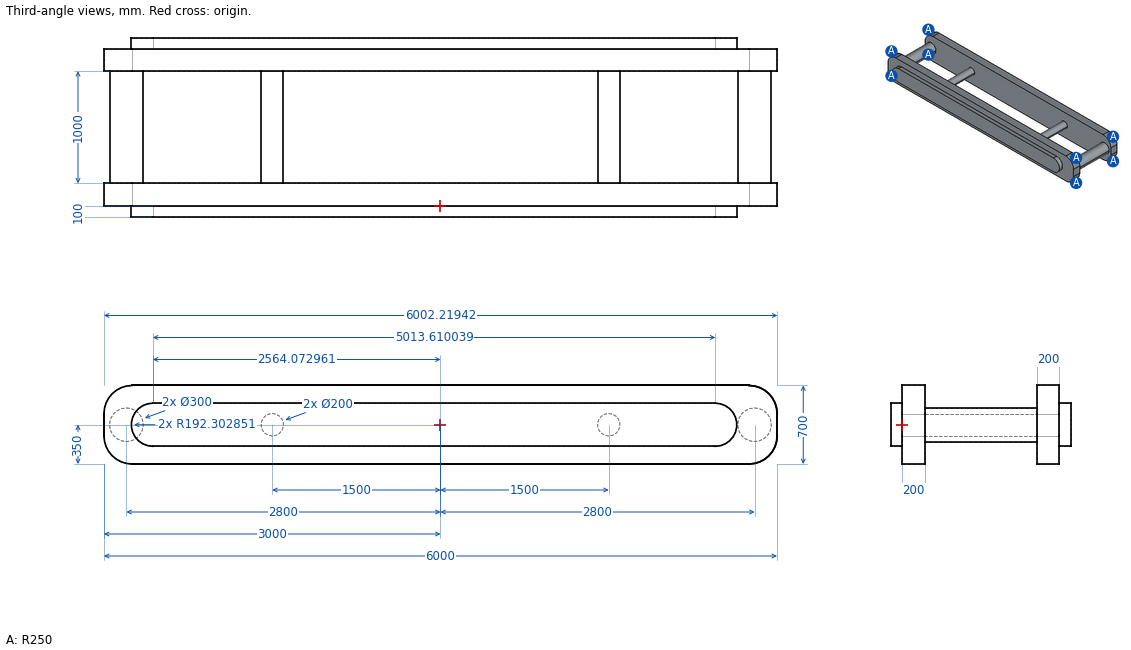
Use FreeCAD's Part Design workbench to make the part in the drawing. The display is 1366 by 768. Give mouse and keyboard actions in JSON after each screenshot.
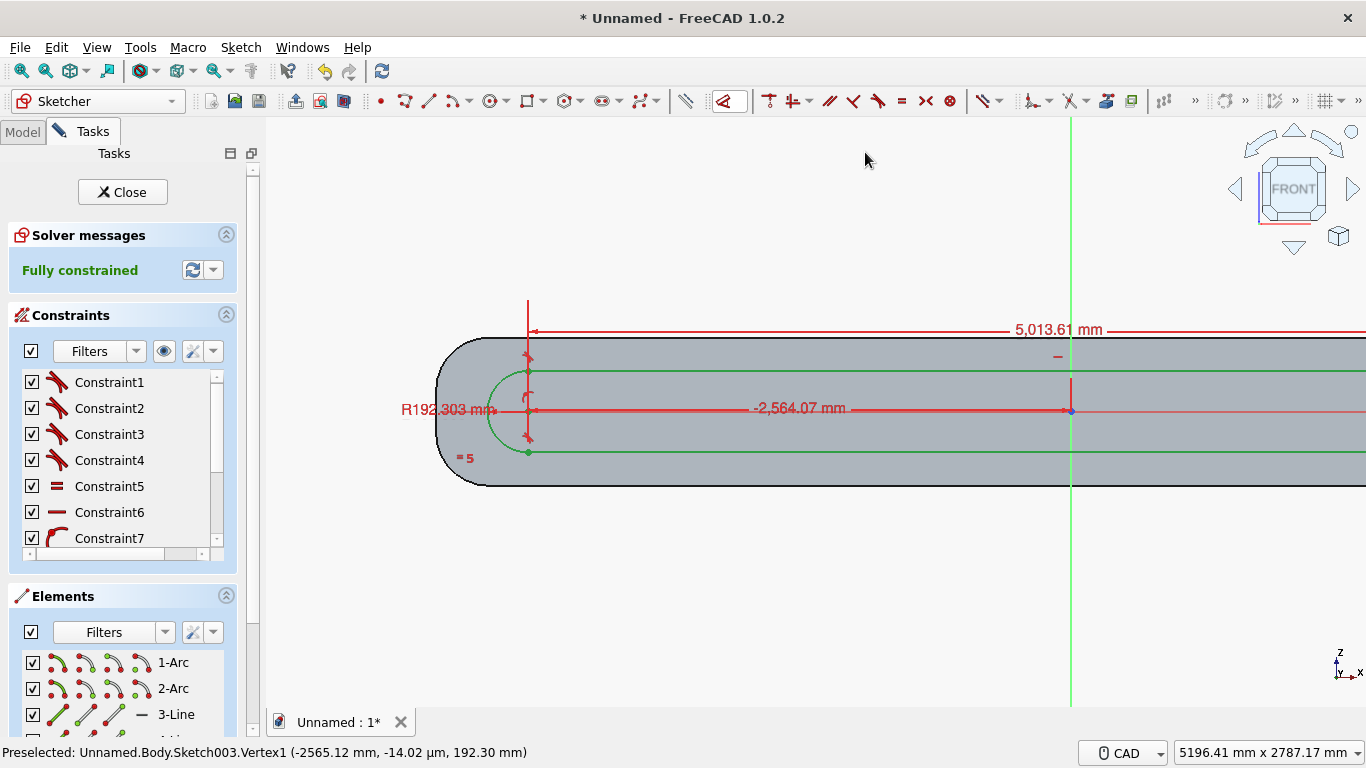
{"action": "left_click", "coordinate": [123, 192]}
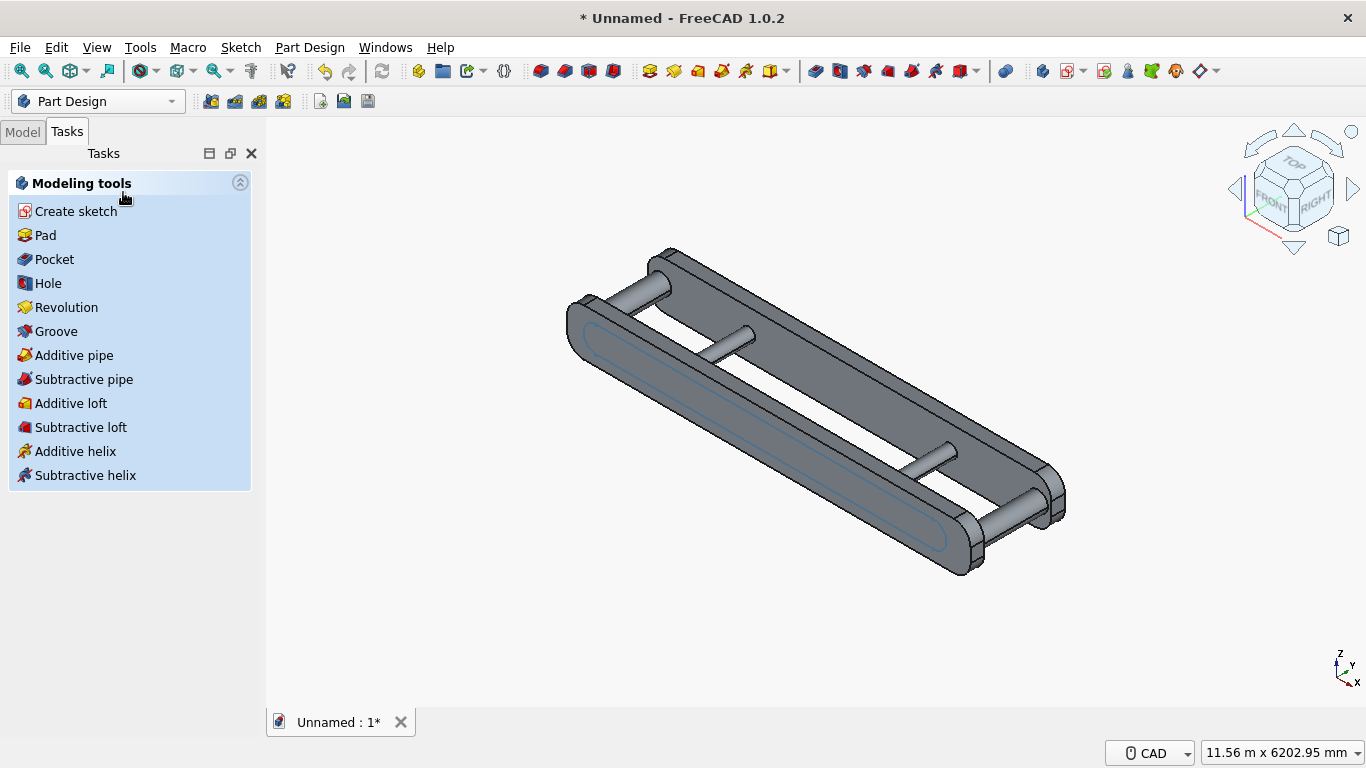
{"action": "left_click", "coordinate": [650, 72]}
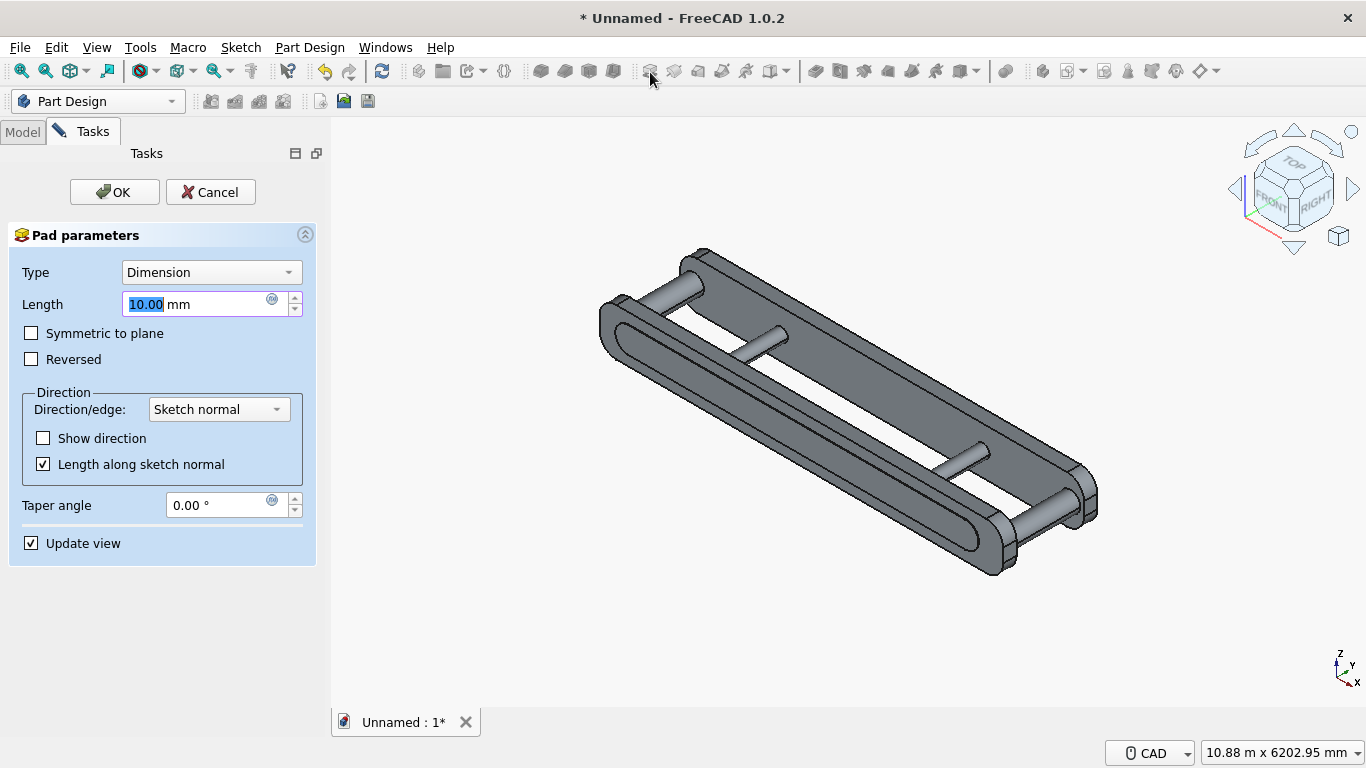
{"action": "type", "text": "100"}
{"action": "key", "text": "Tab"}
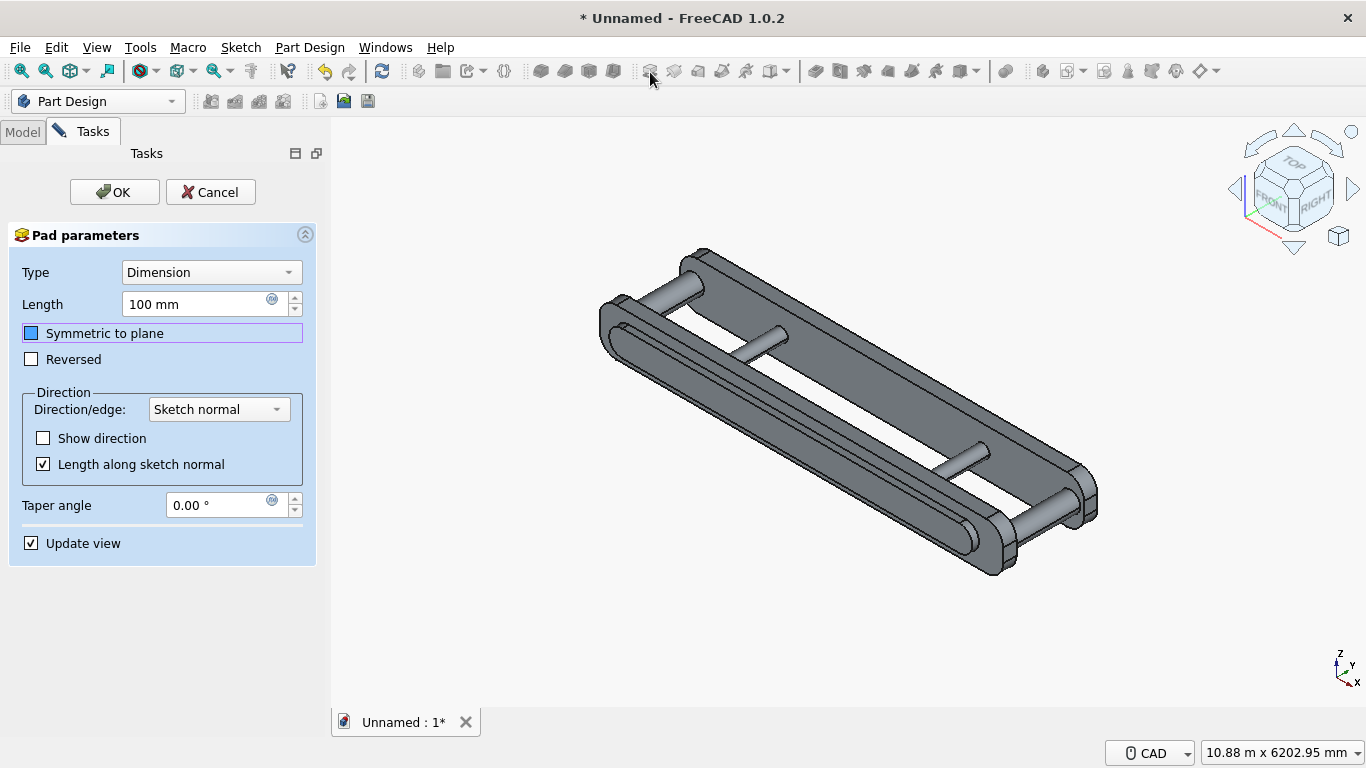
{"action": "left_click", "coordinate": [115, 192]}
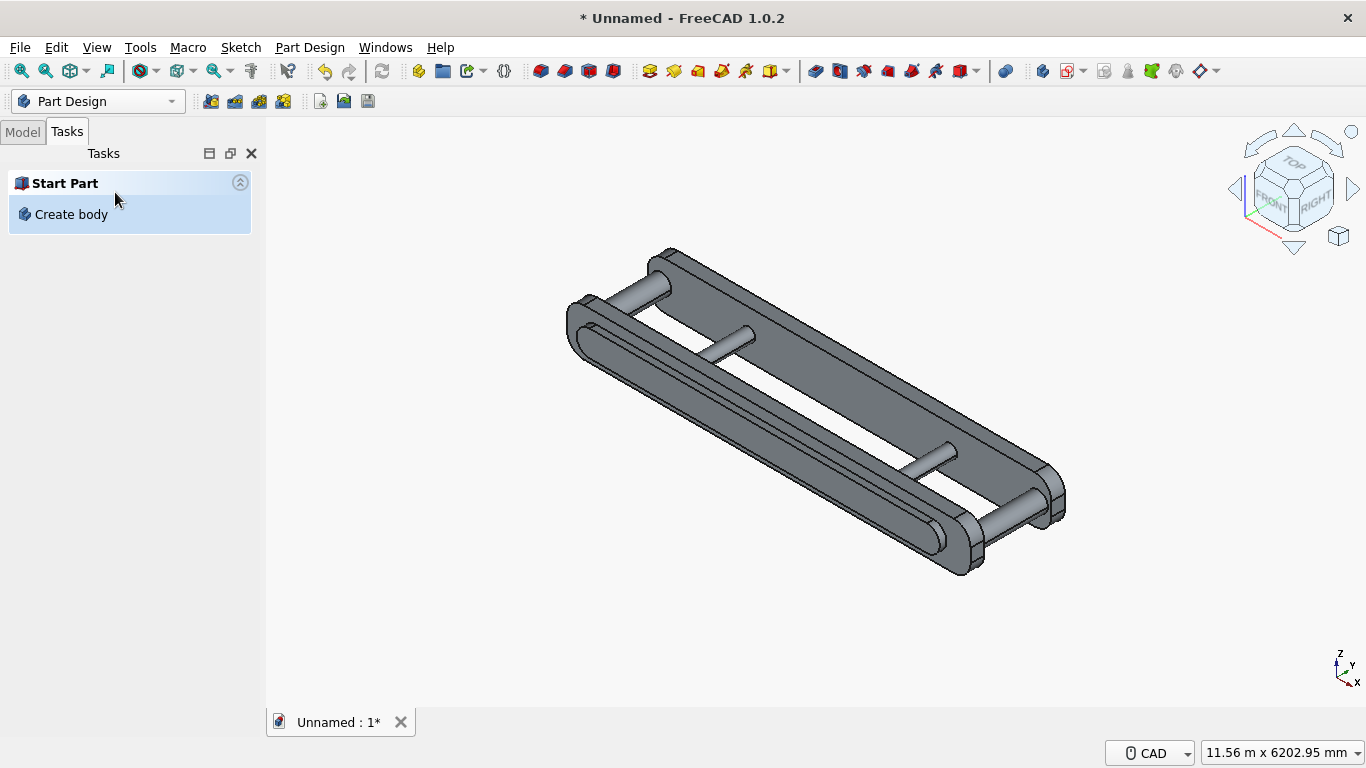
{"action": "left_click", "coordinate": [23, 131]}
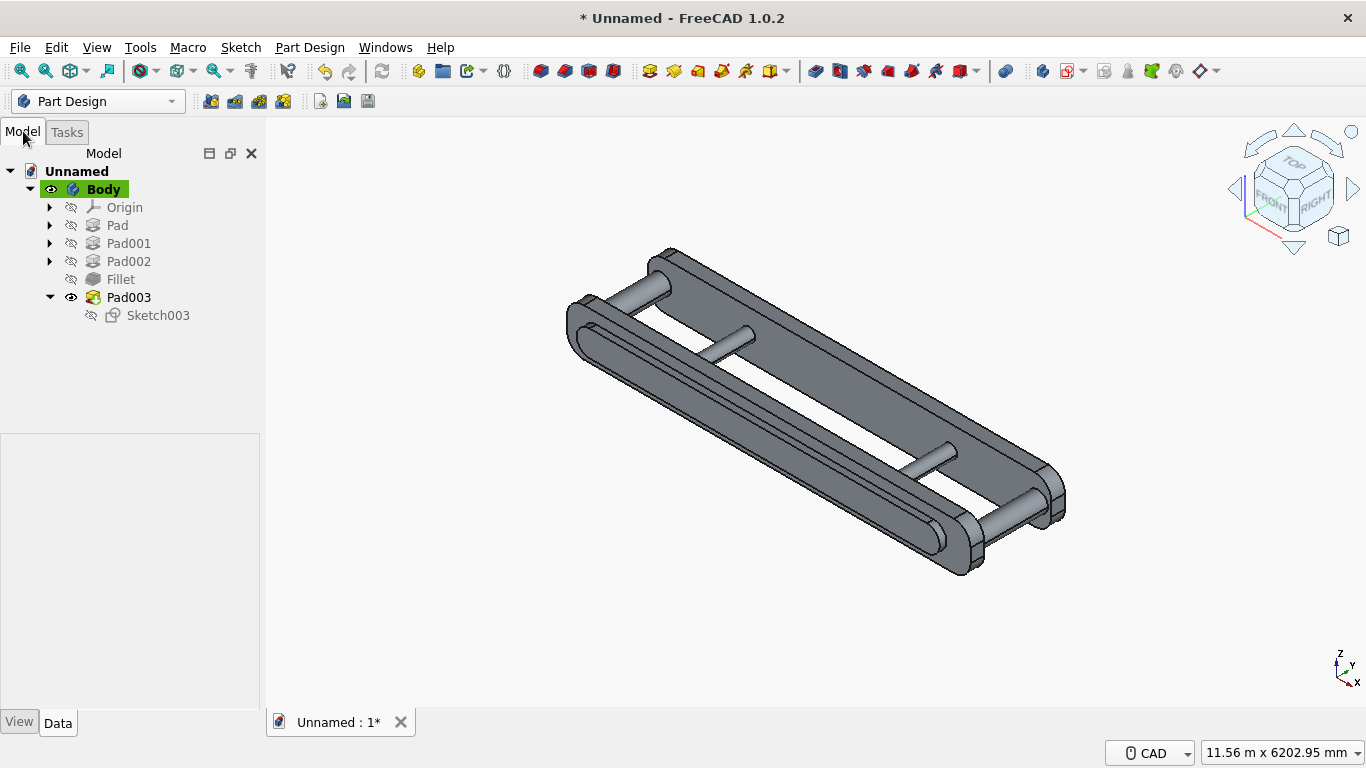
{"action": "left_click", "coordinate": [50, 207]}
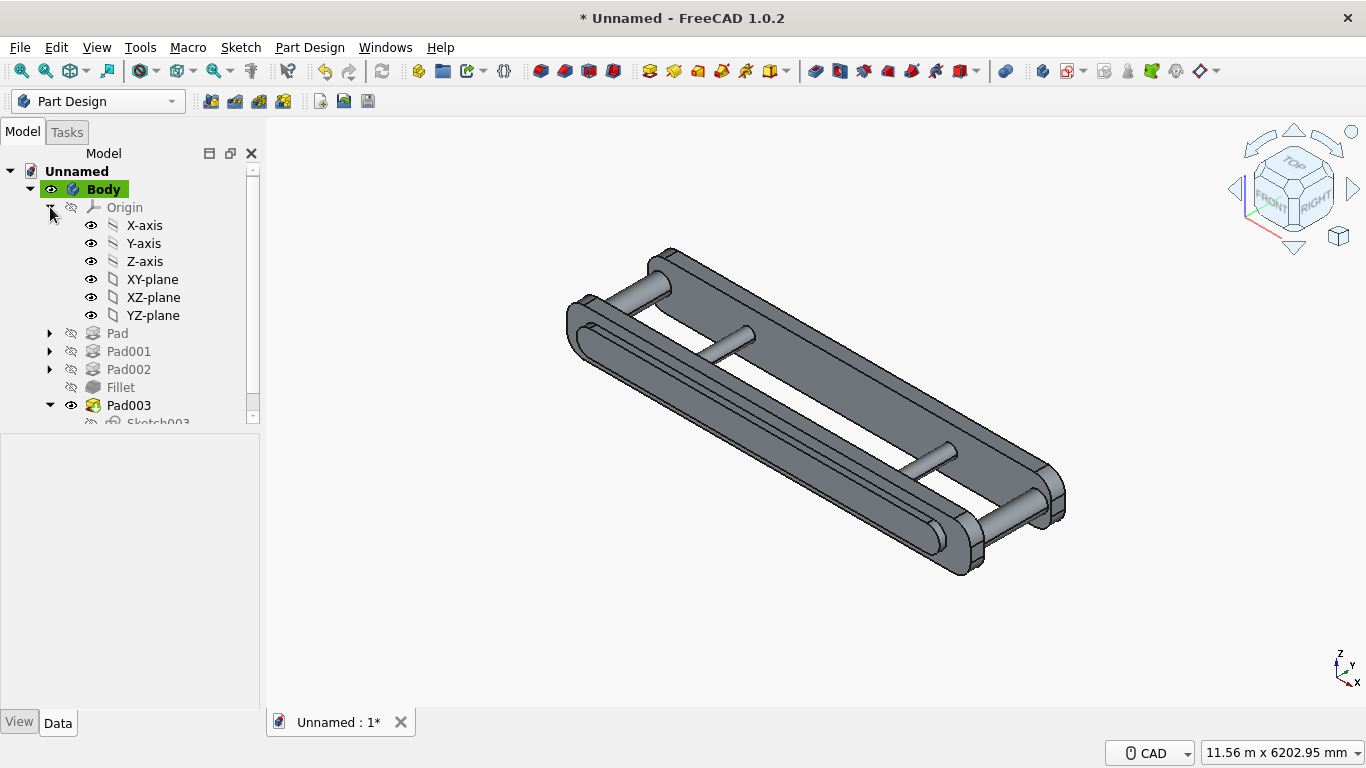
{"action": "left_click", "coordinate": [136, 297]}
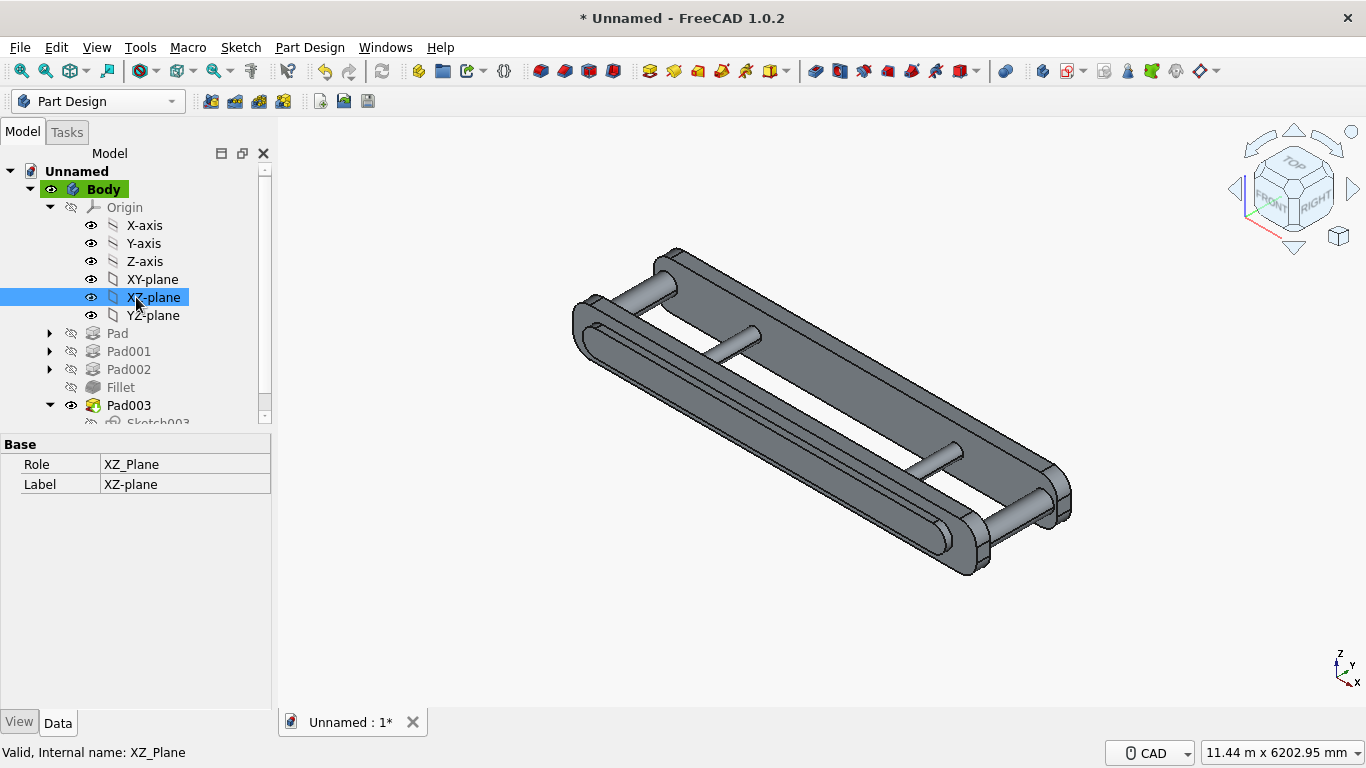
{"action": "left_click", "coordinate": [1200, 72]}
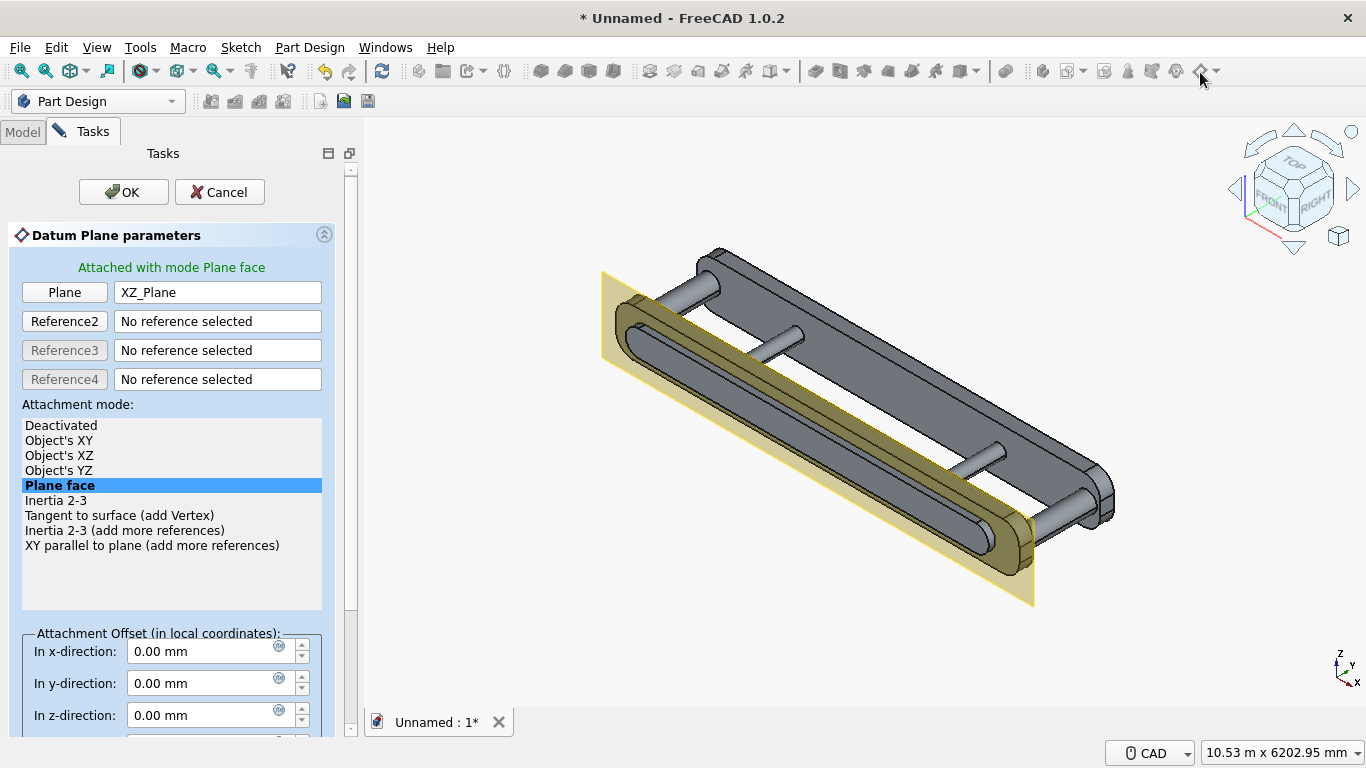
{"action": "triple_click", "coordinate": [210, 715]}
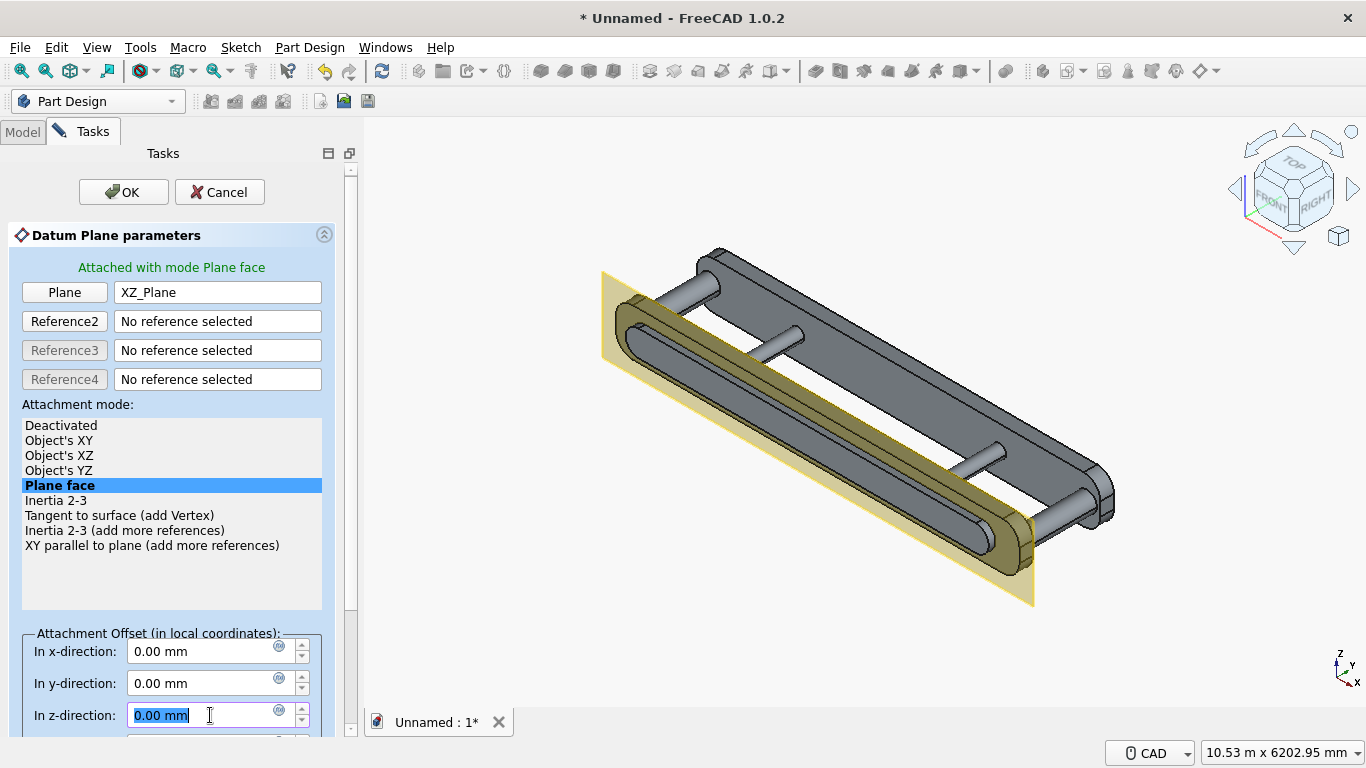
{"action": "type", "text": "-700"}
{"action": "key", "text": "Tab"}